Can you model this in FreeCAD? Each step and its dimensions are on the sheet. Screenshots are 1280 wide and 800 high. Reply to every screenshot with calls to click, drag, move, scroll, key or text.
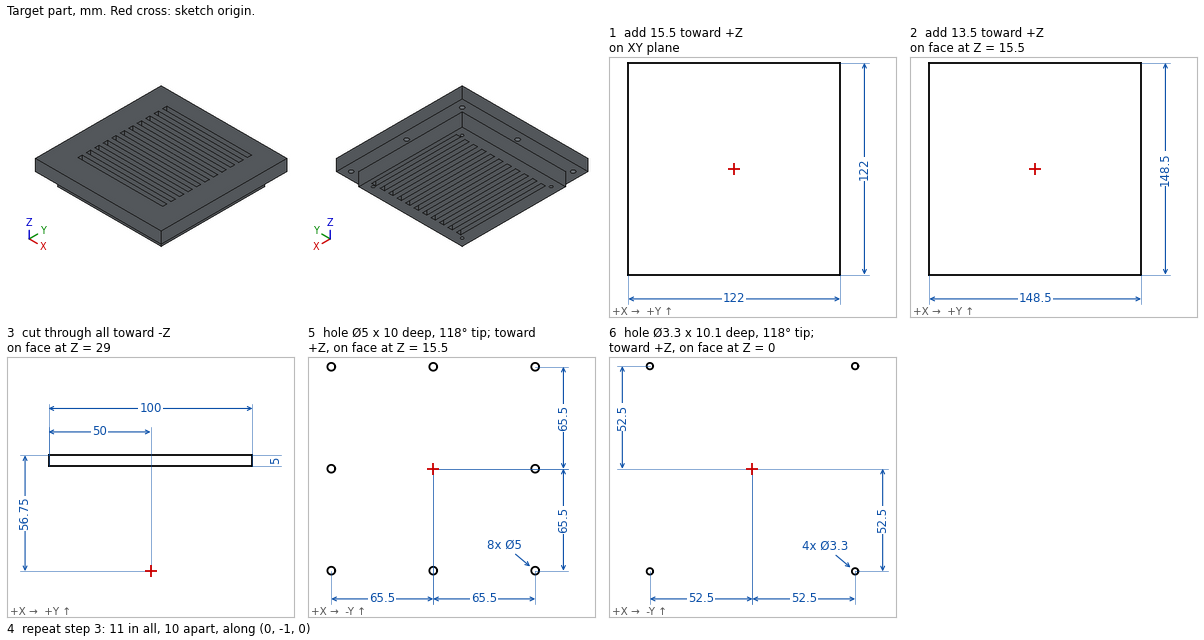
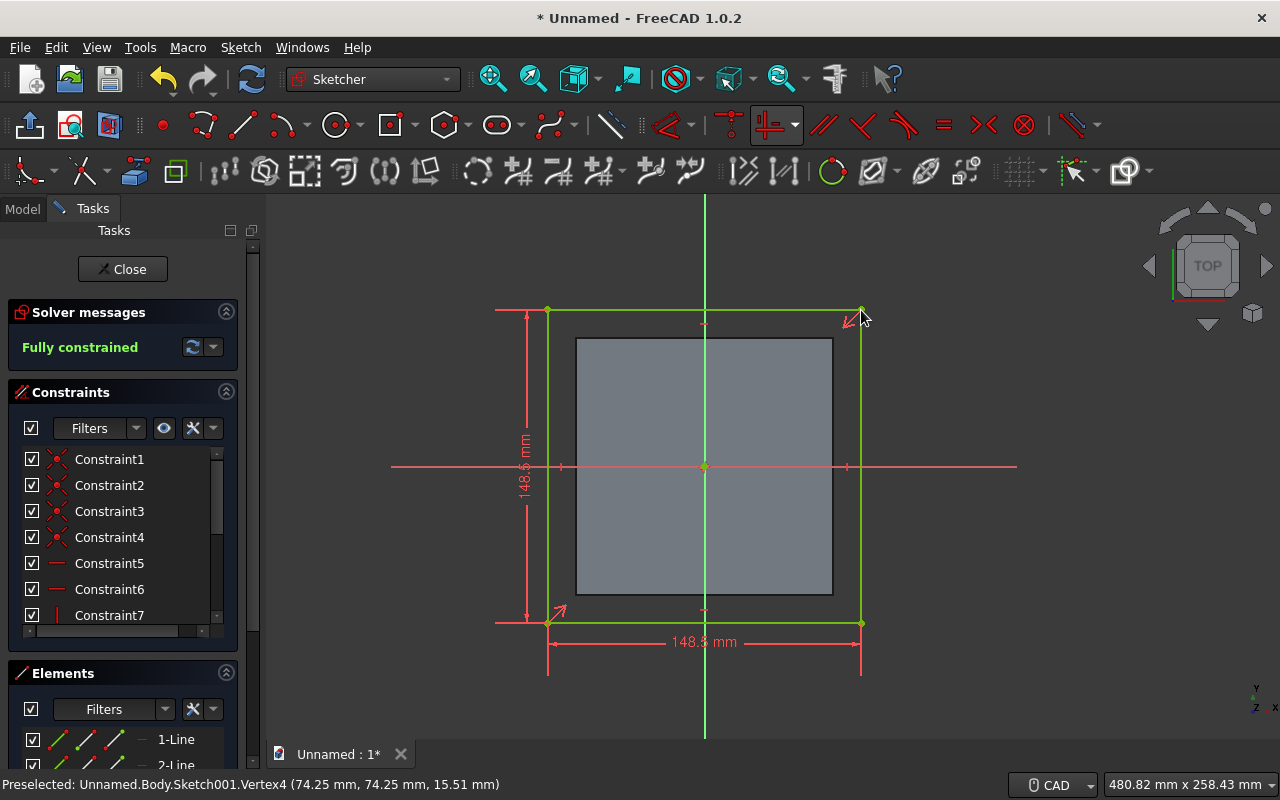
click(123, 269)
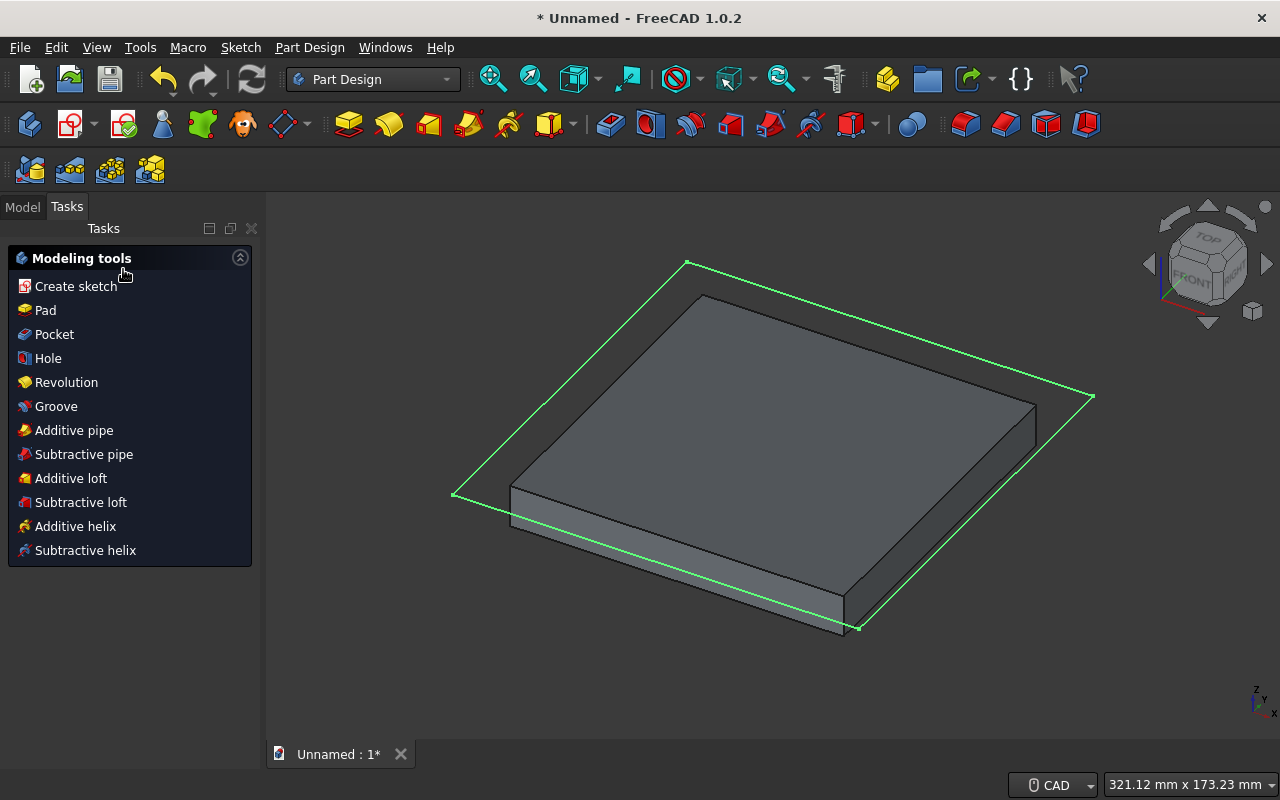
click(350, 124)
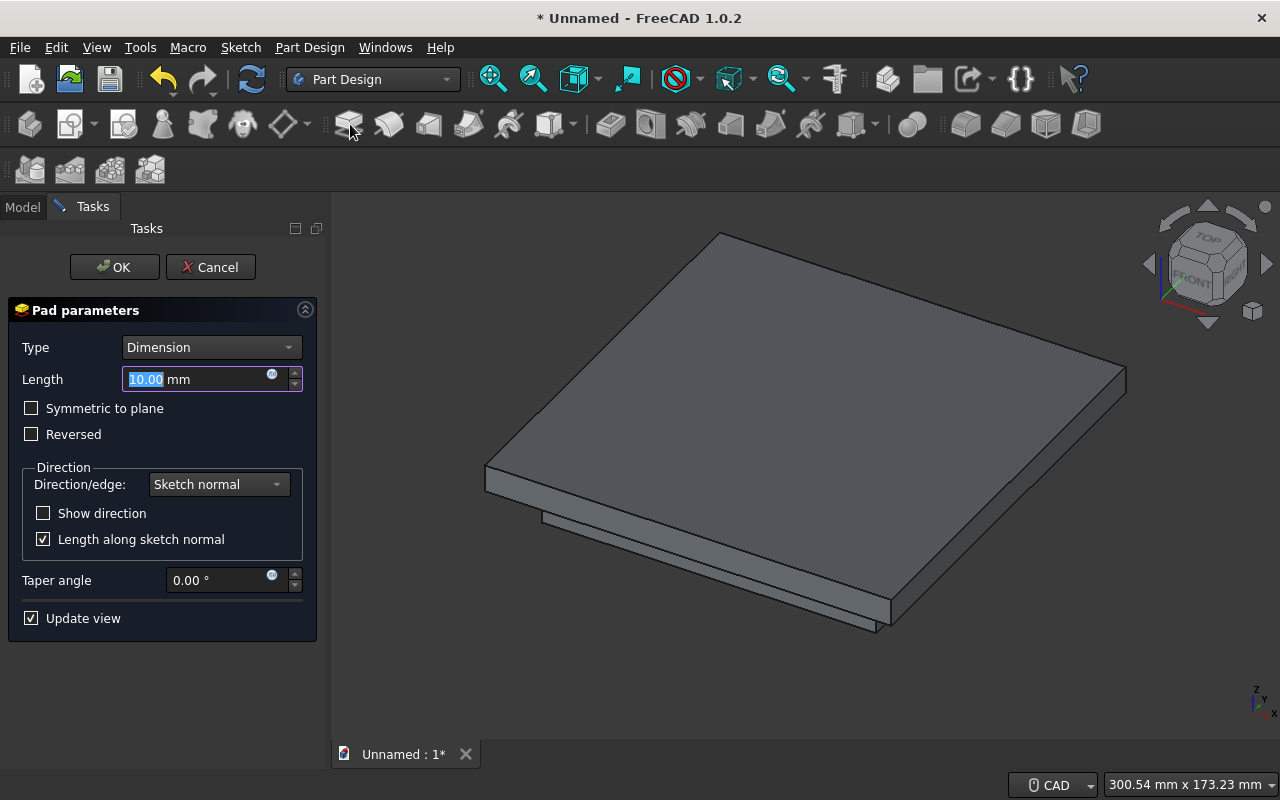
text(13.5)
key(Tab)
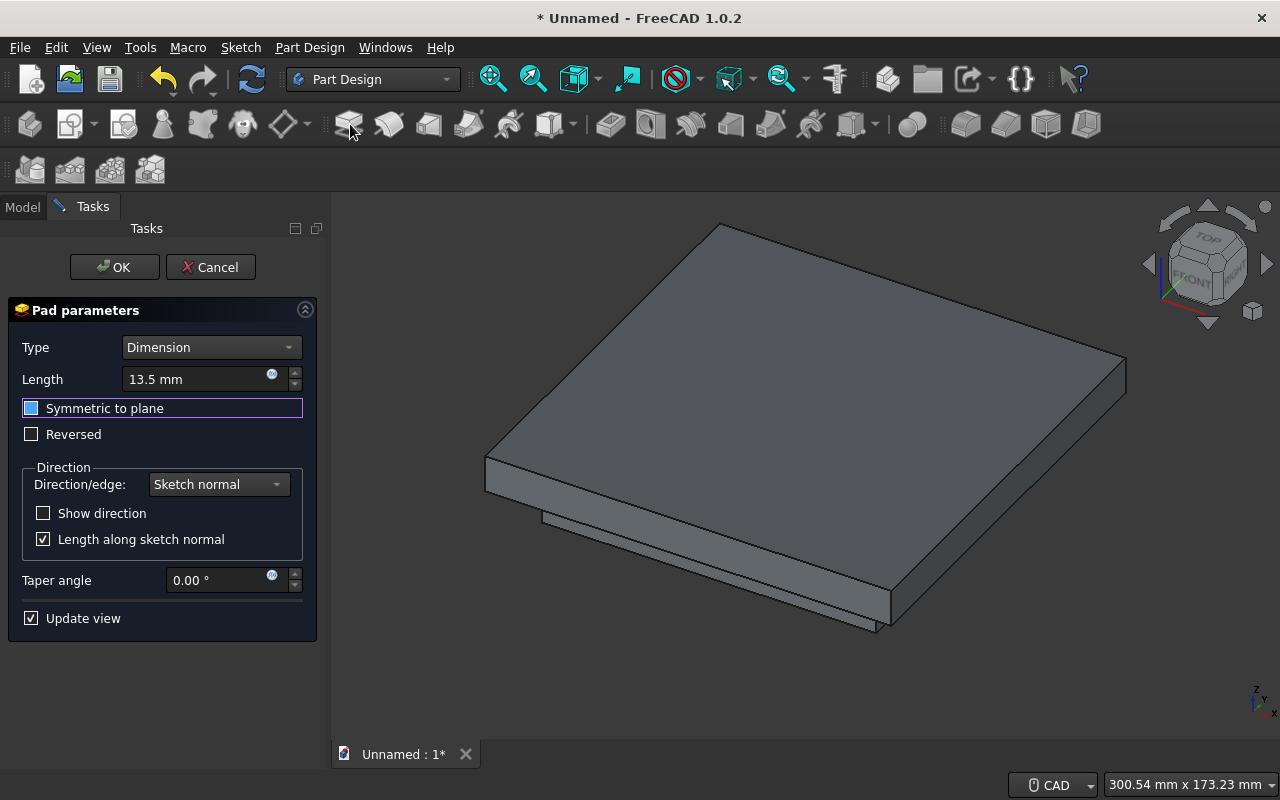
click(115, 267)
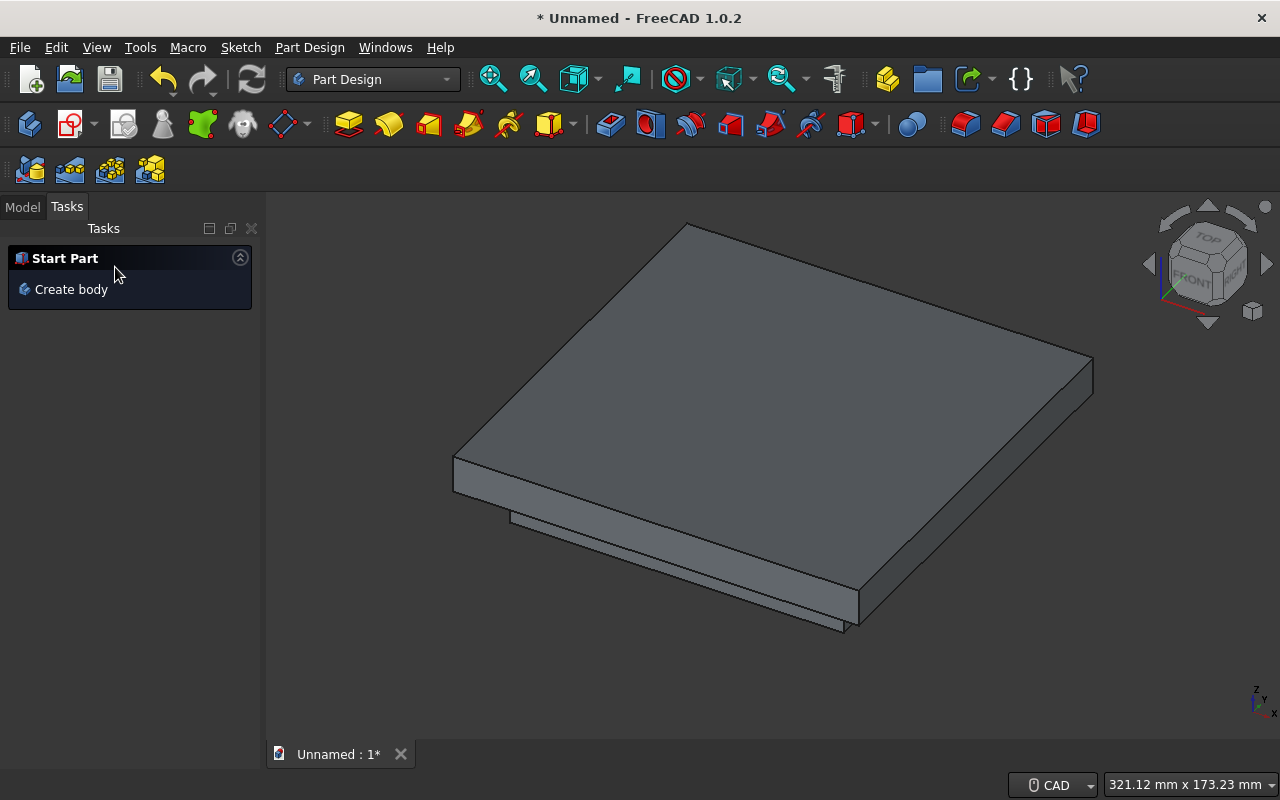
click(773, 406)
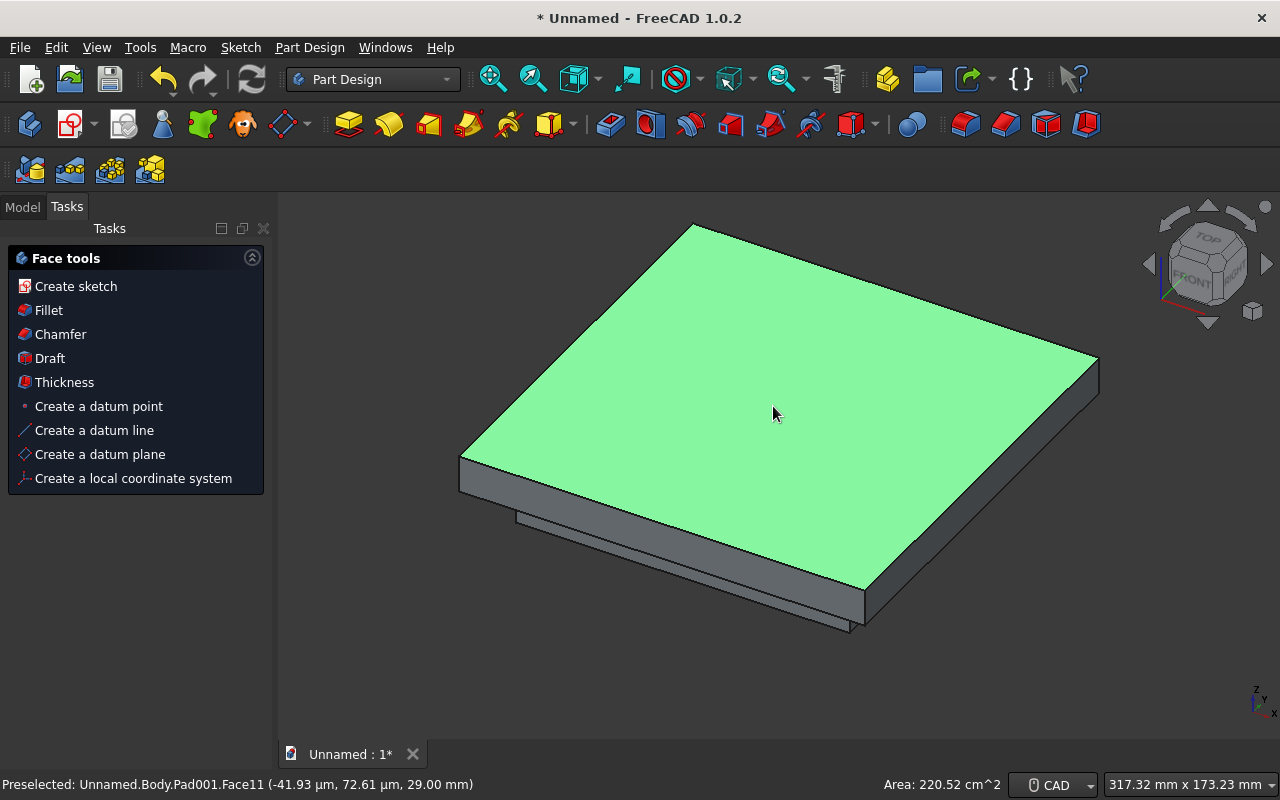
click(70, 124)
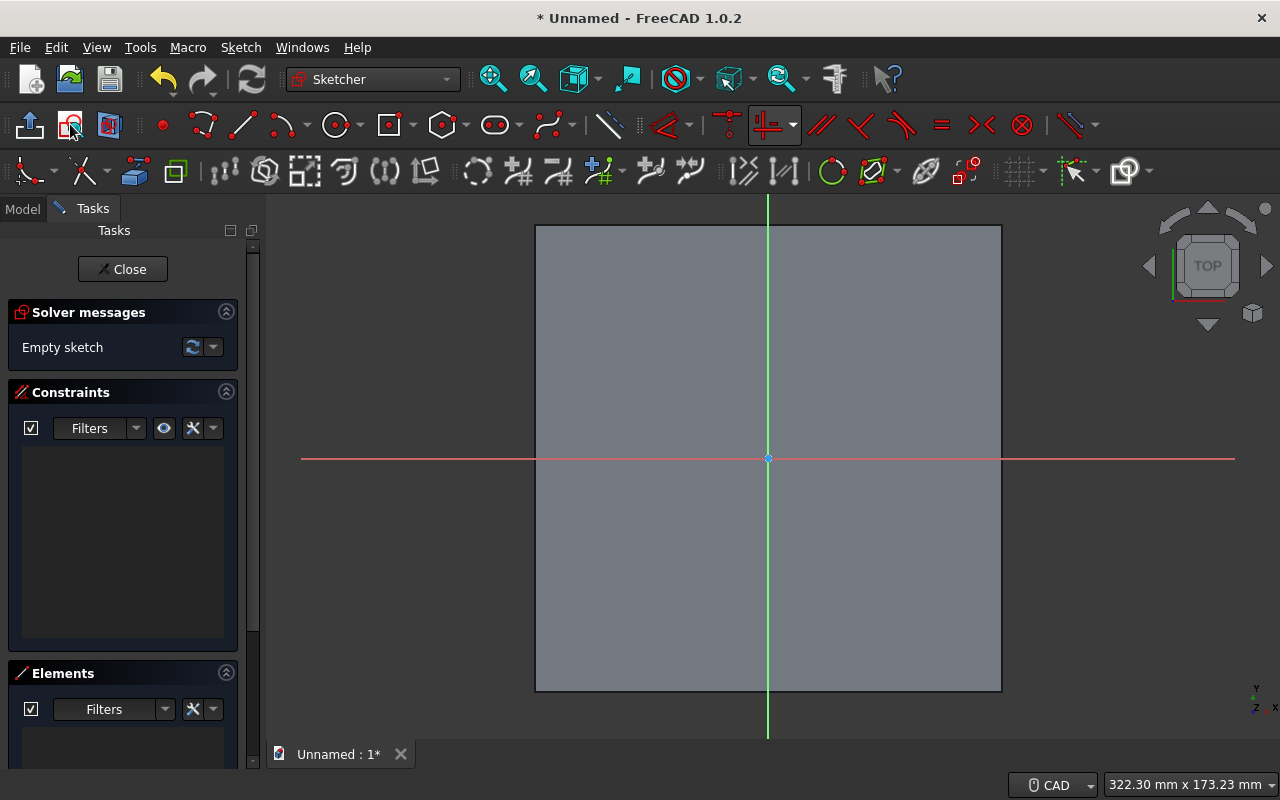
scroll(846, 251, up, 3)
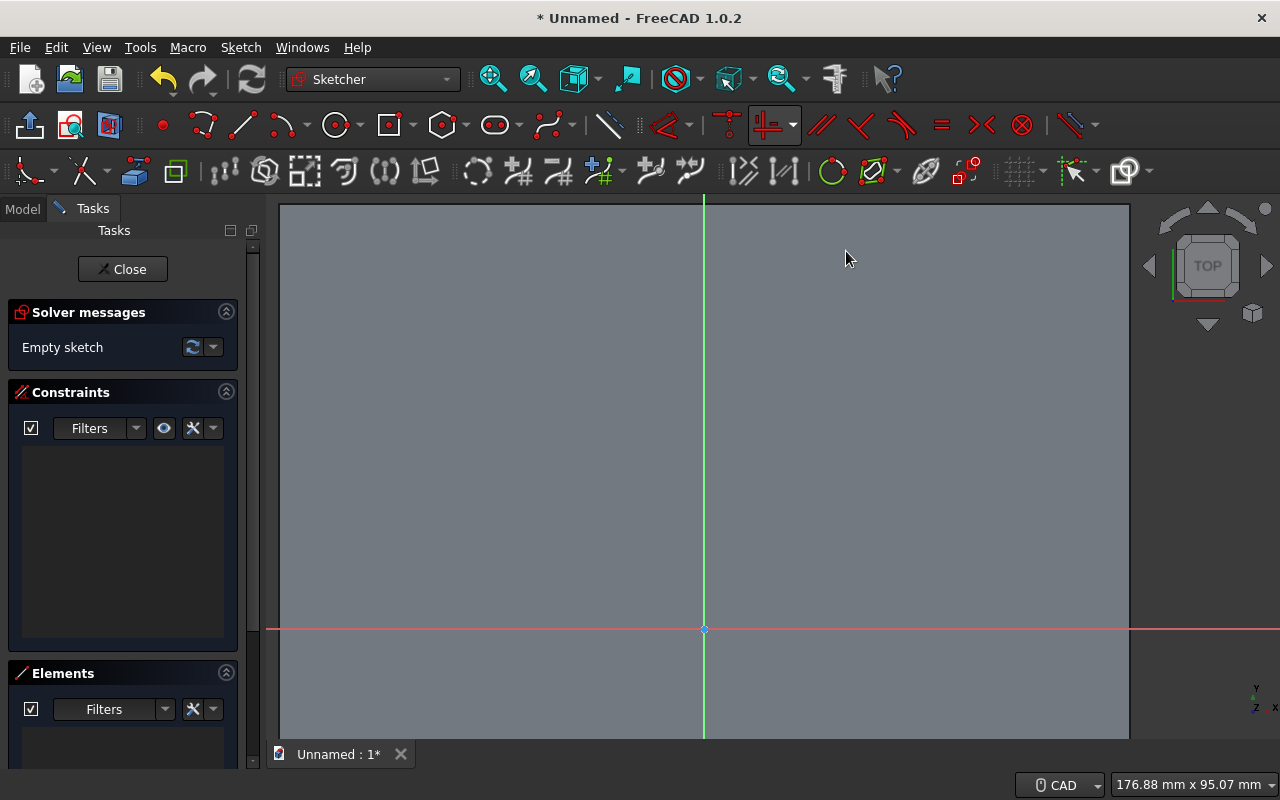
click(416, 126)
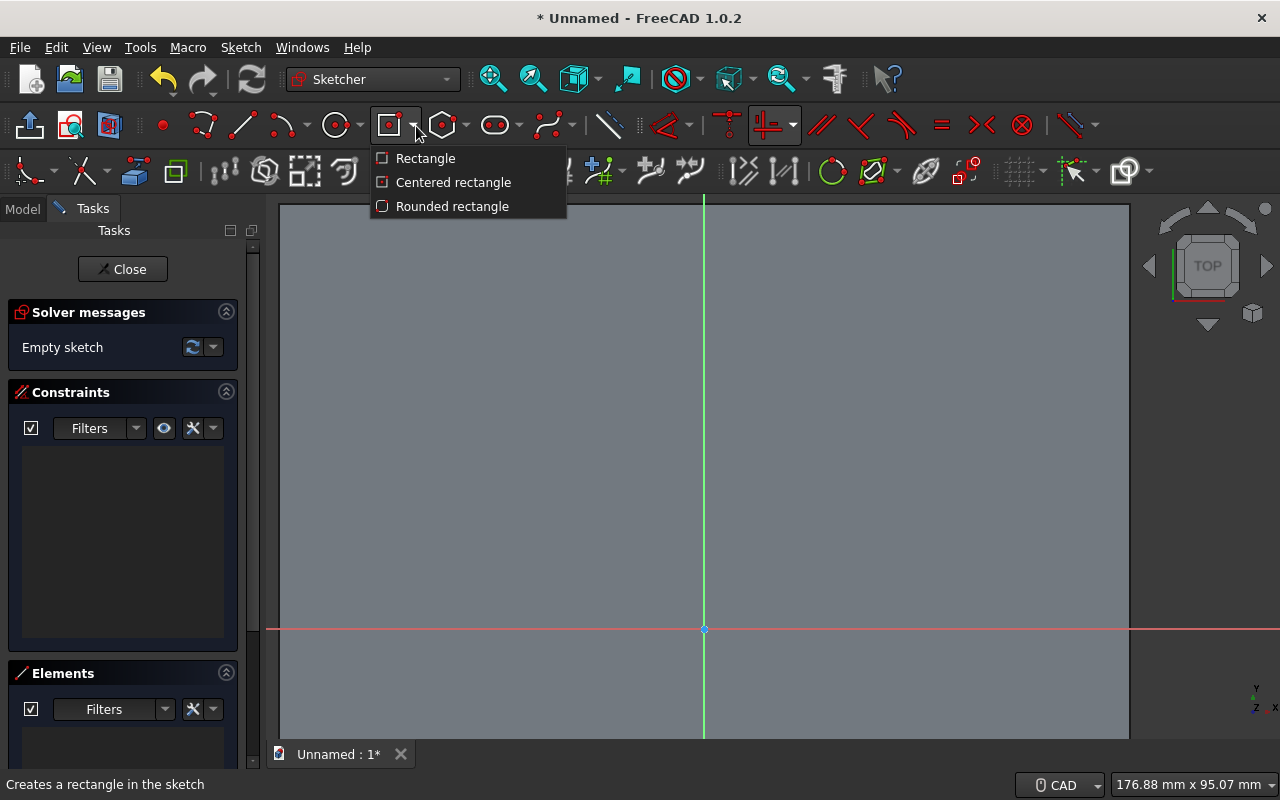
click(468, 158)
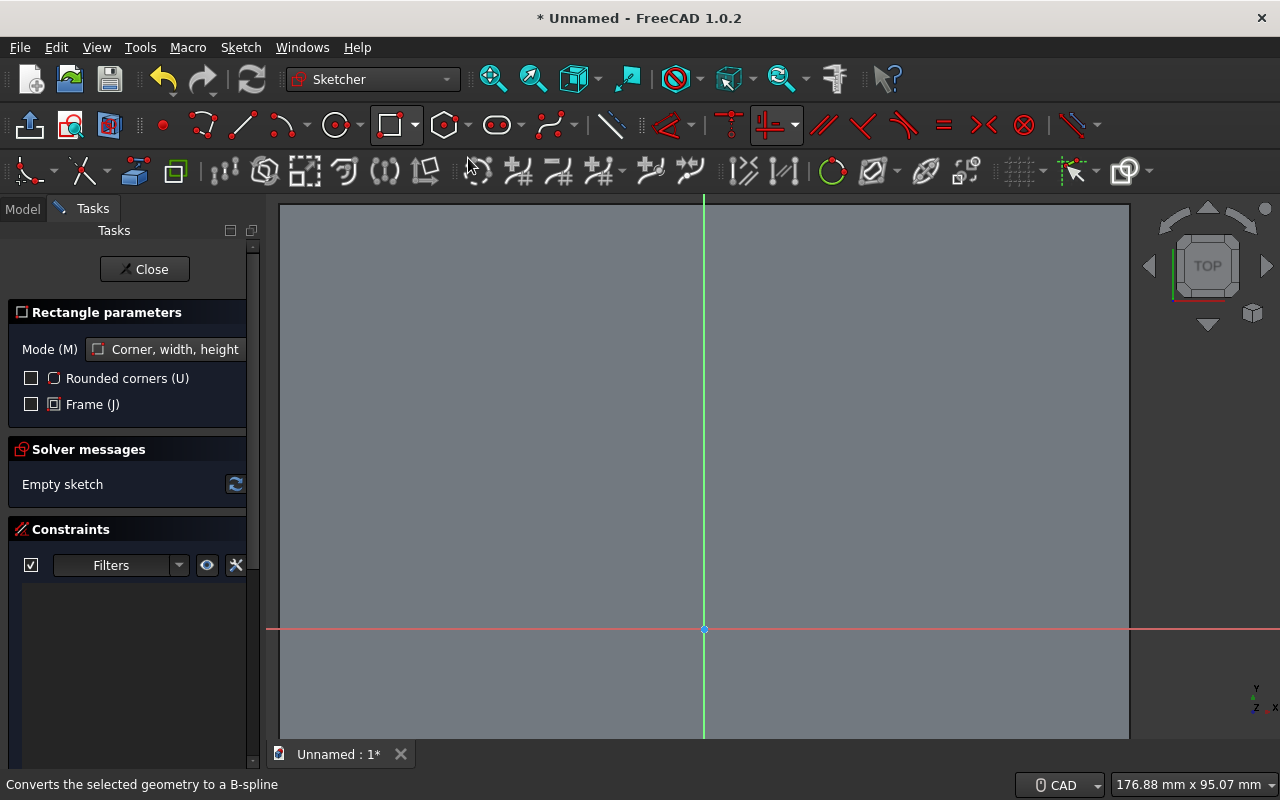
click(418, 304)
move(991, 333)